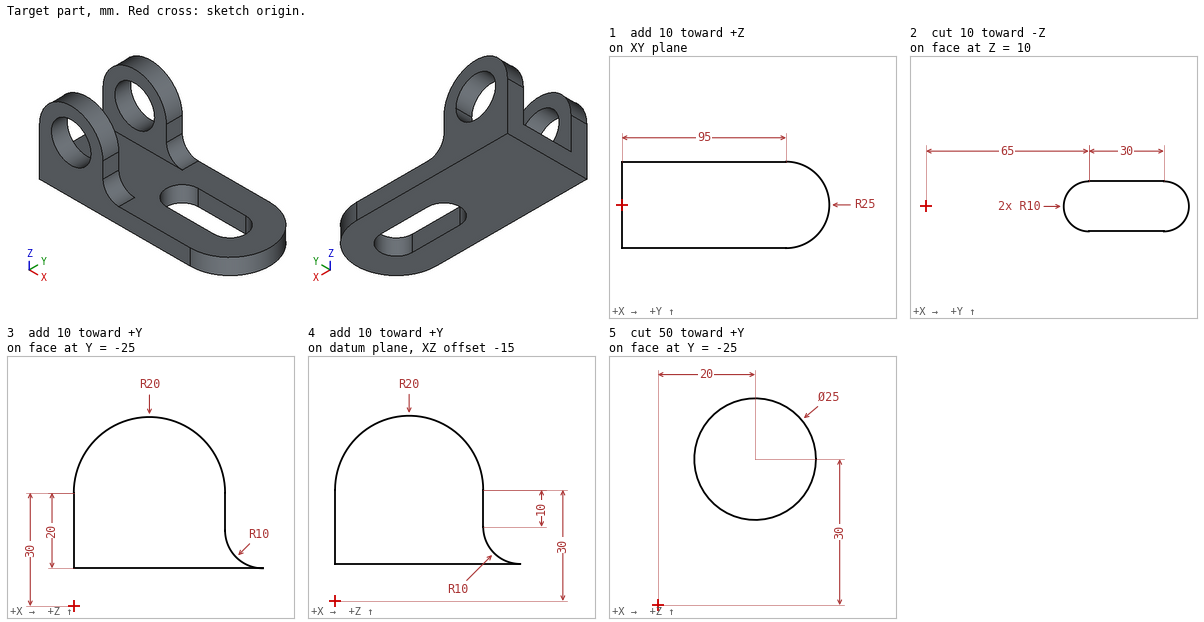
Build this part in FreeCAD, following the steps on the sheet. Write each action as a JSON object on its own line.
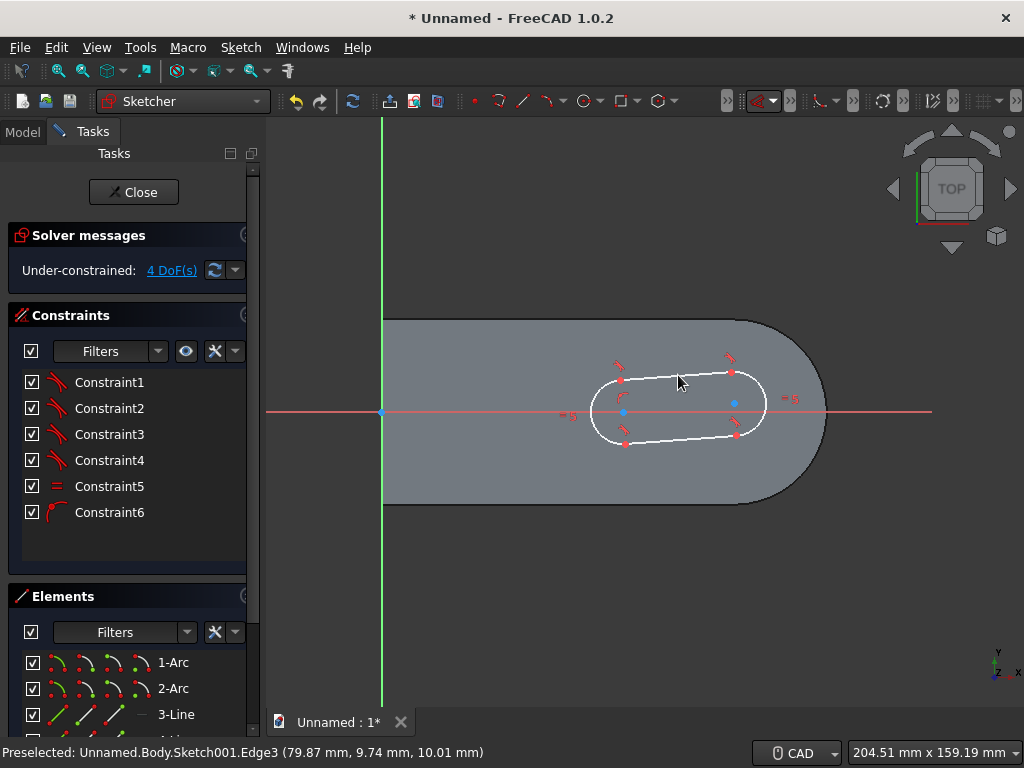
{"action": "left_click", "coordinate": [654, 378]}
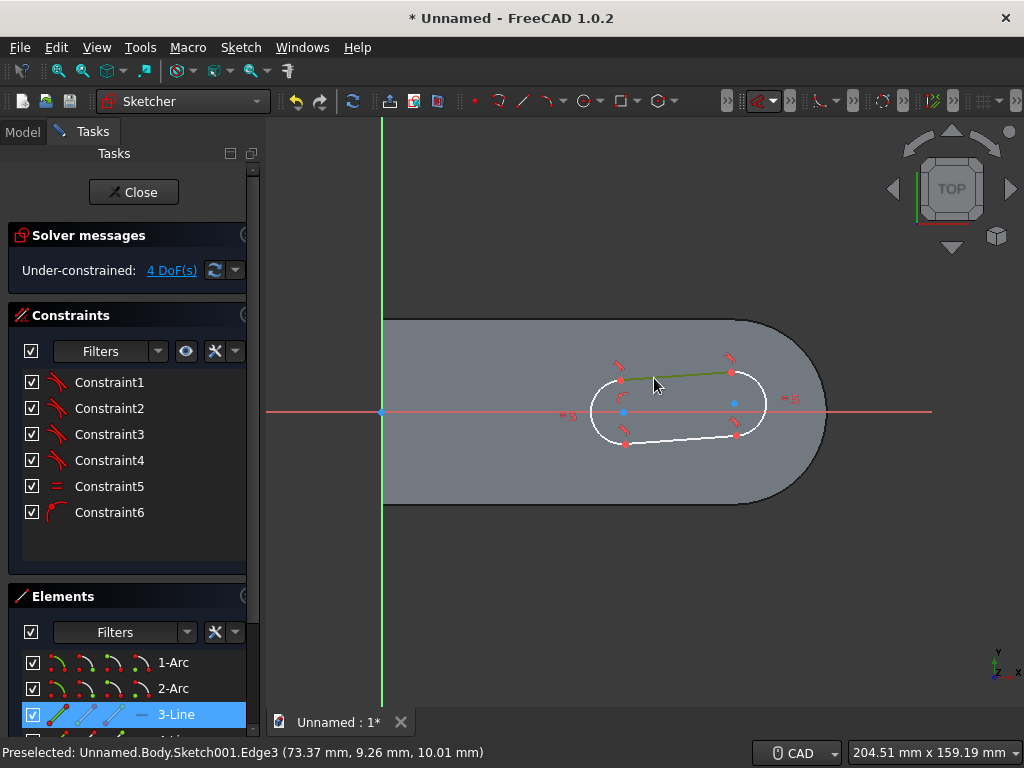
{"action": "key", "text": "h"}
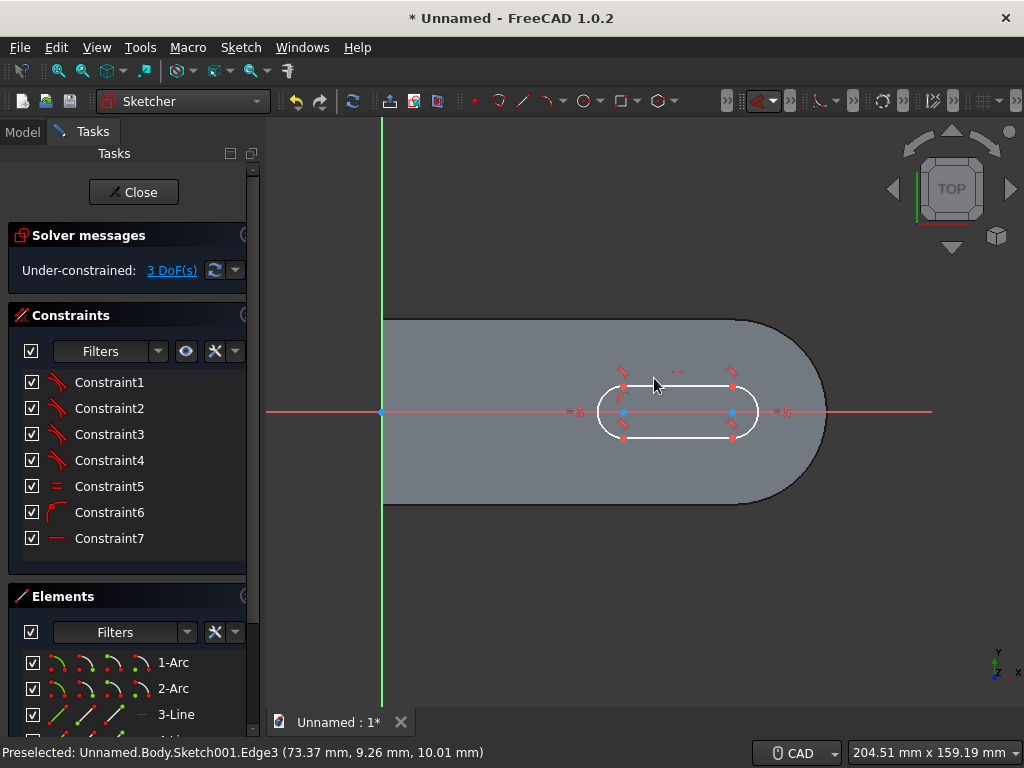
{"action": "left_click", "coordinate": [603, 397]}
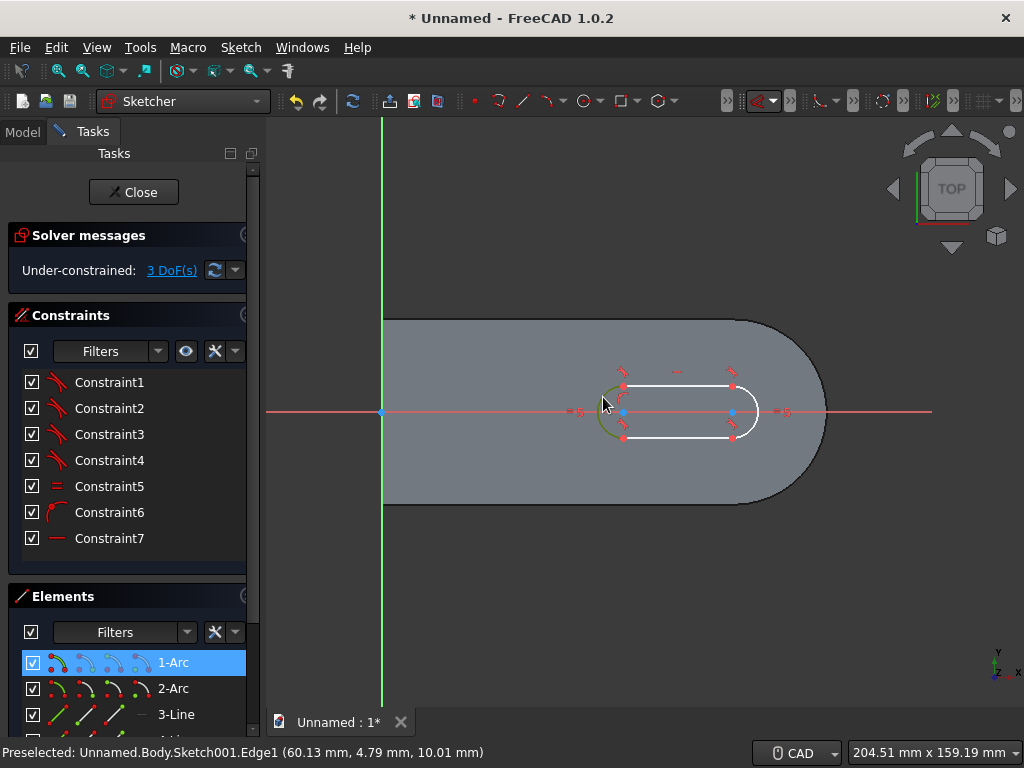
{"action": "left_click", "coordinate": [776, 102]}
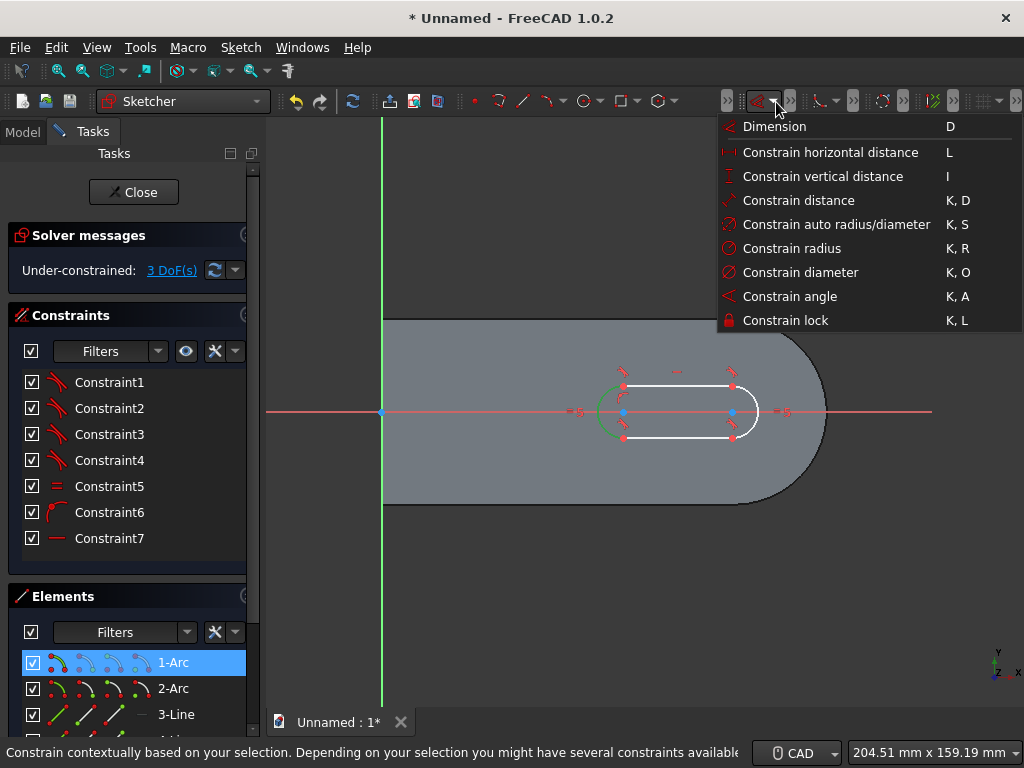
{"action": "left_click", "coordinate": [870, 248]}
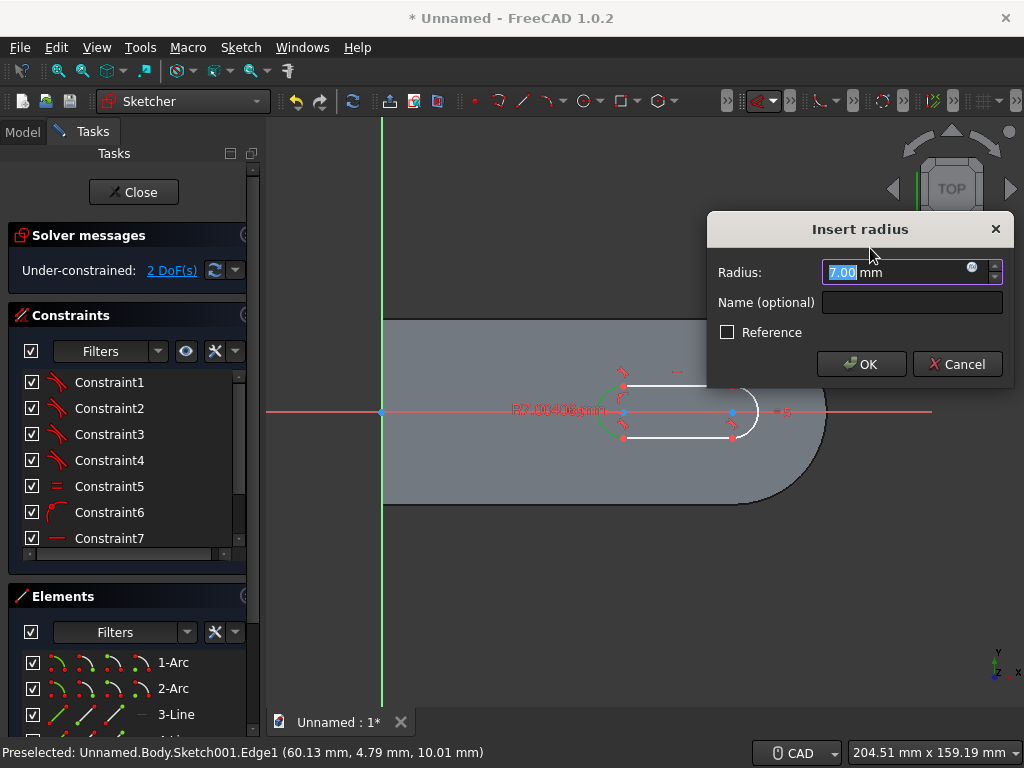
{"action": "type", "text": "10"}
{"action": "key", "text": "Return"}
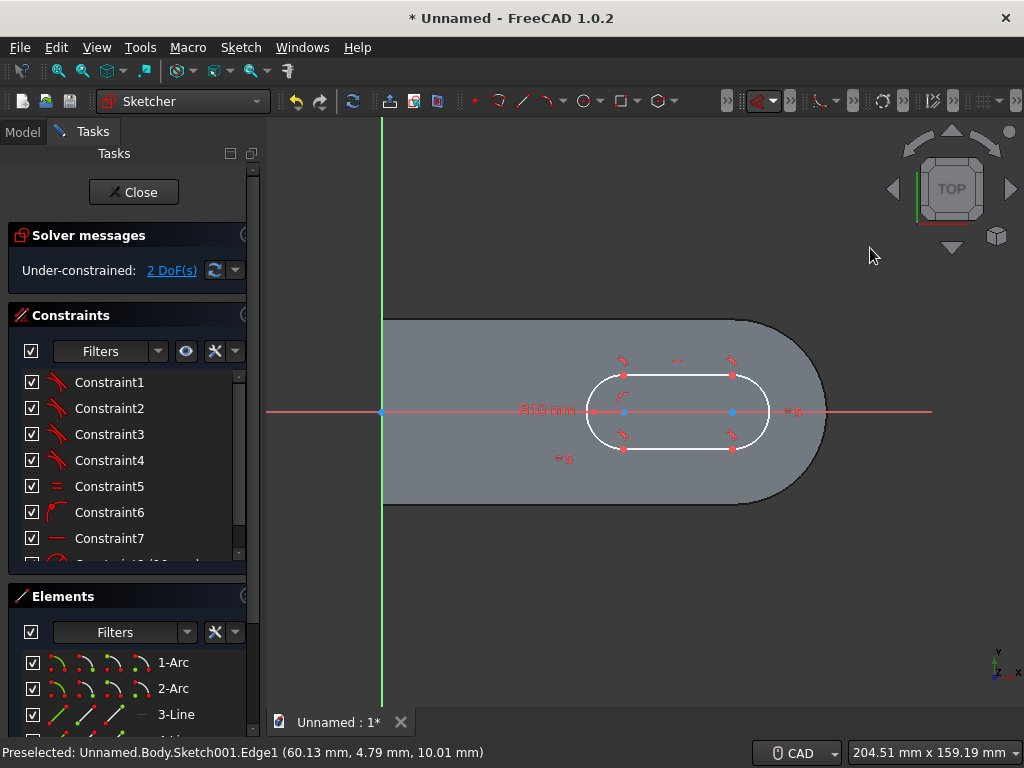
{"action": "left_click", "coordinate": [656, 375]}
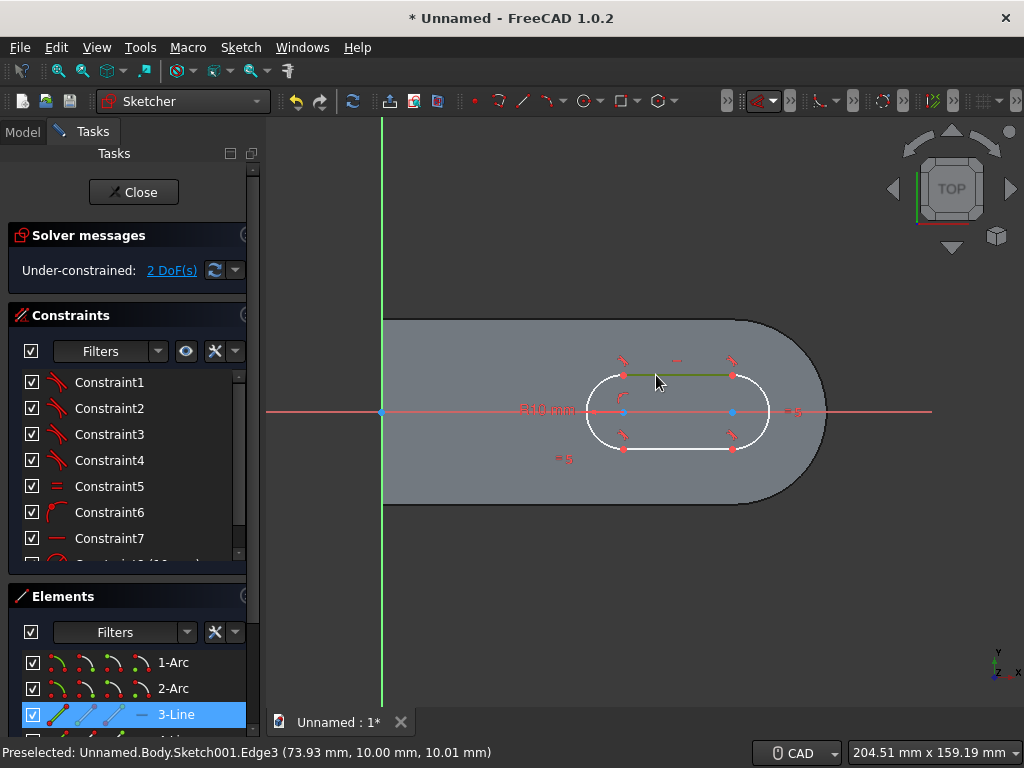
{"action": "left_click", "coordinate": [776, 102]}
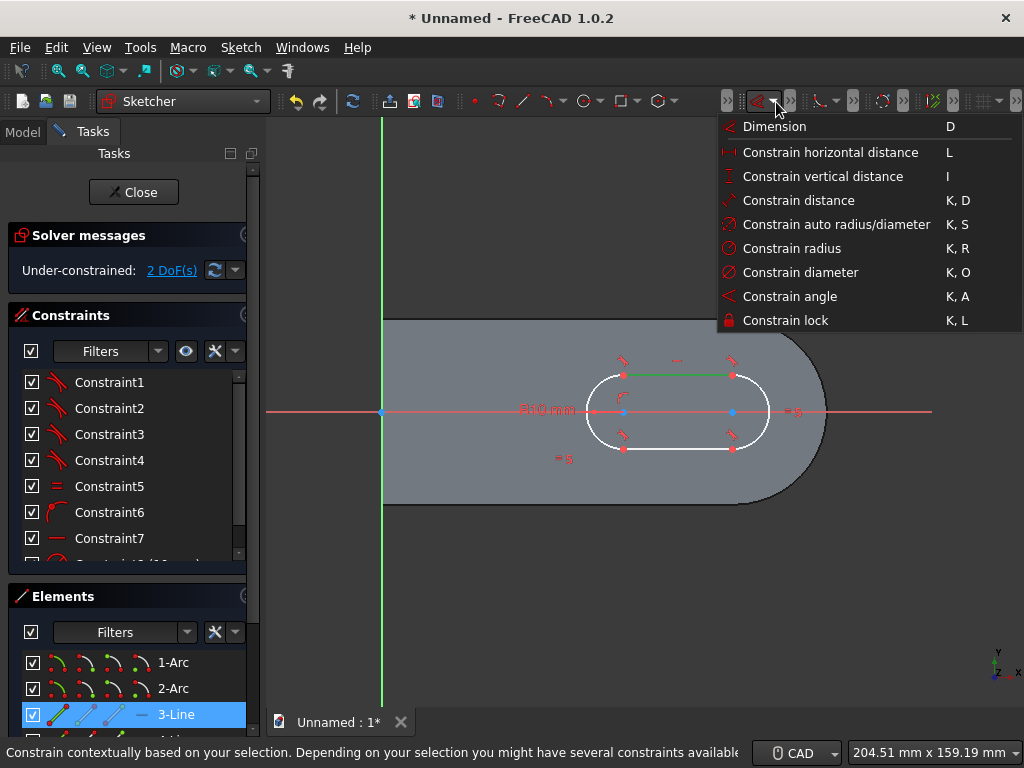
{"action": "left_click", "coordinate": [870, 152]}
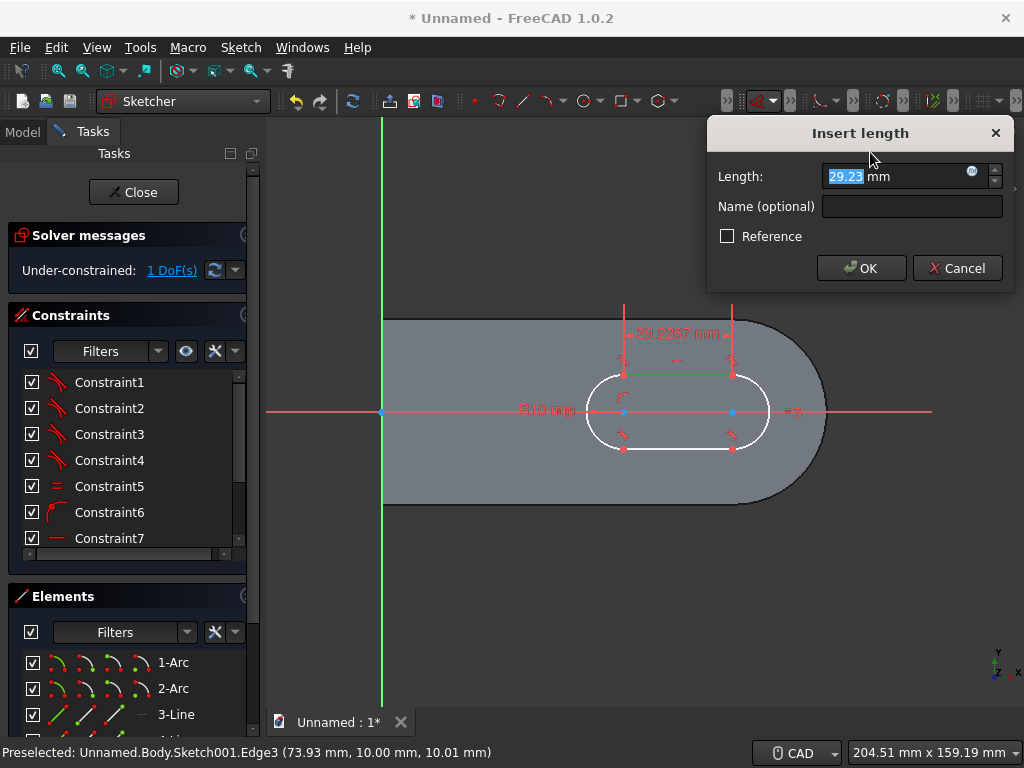
{"action": "type", "text": "30"}
{"action": "key", "text": "Return"}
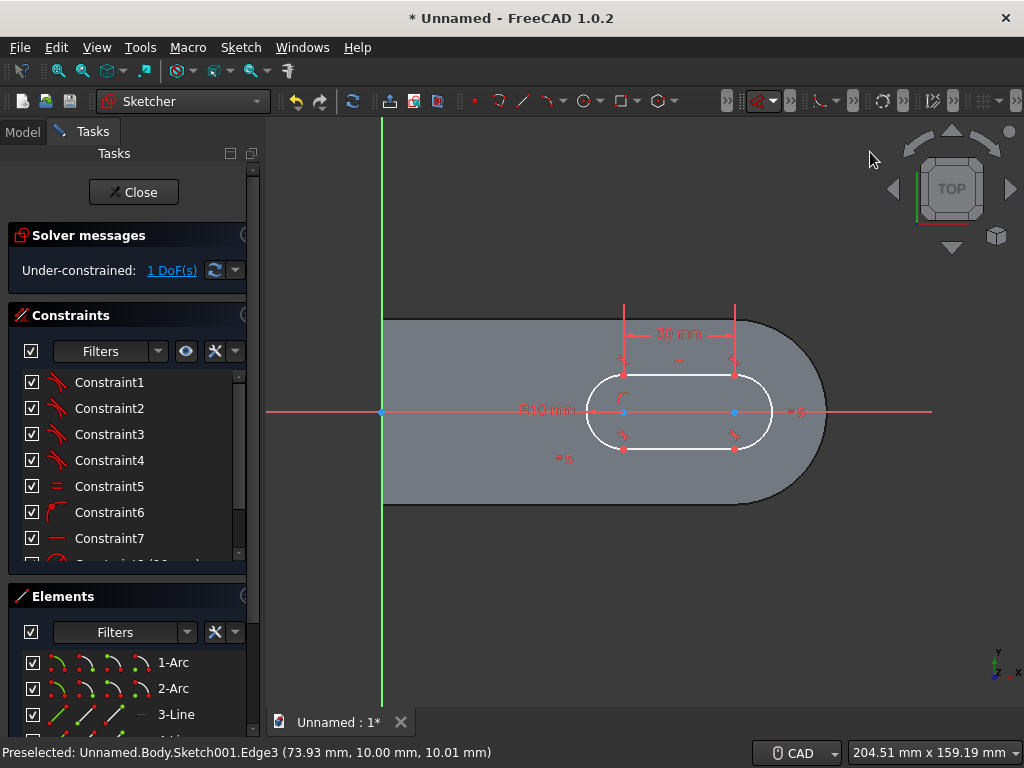
{"action": "left_click", "coordinate": [624, 375]}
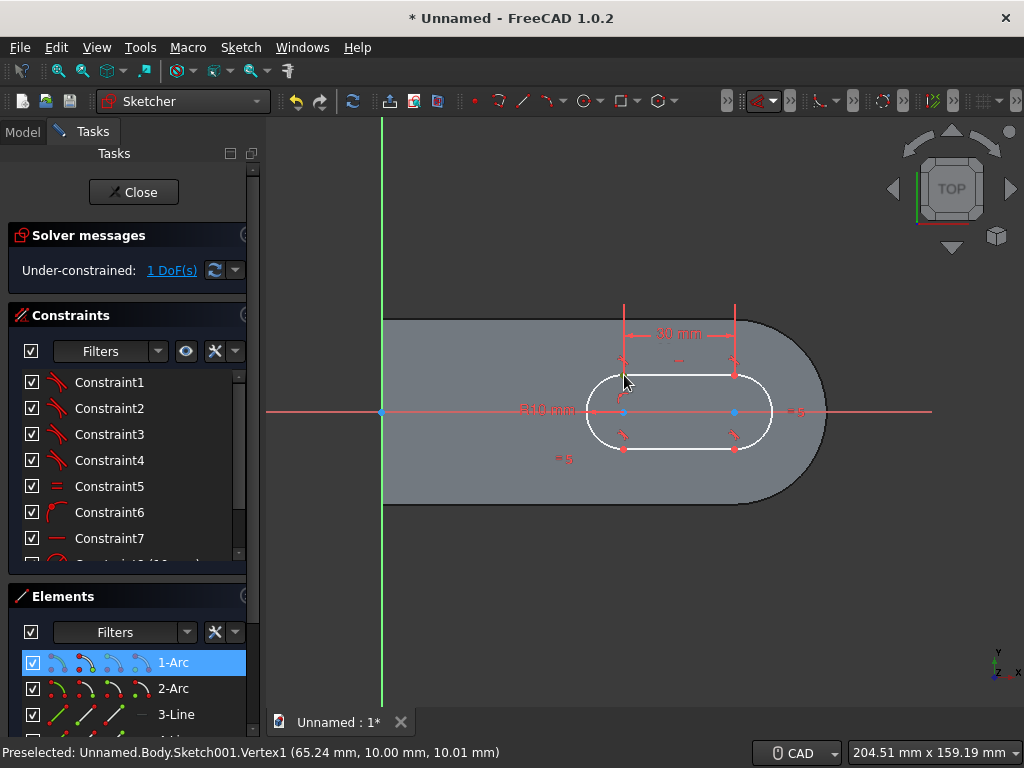
{"action": "left_click", "coordinate": [776, 102]}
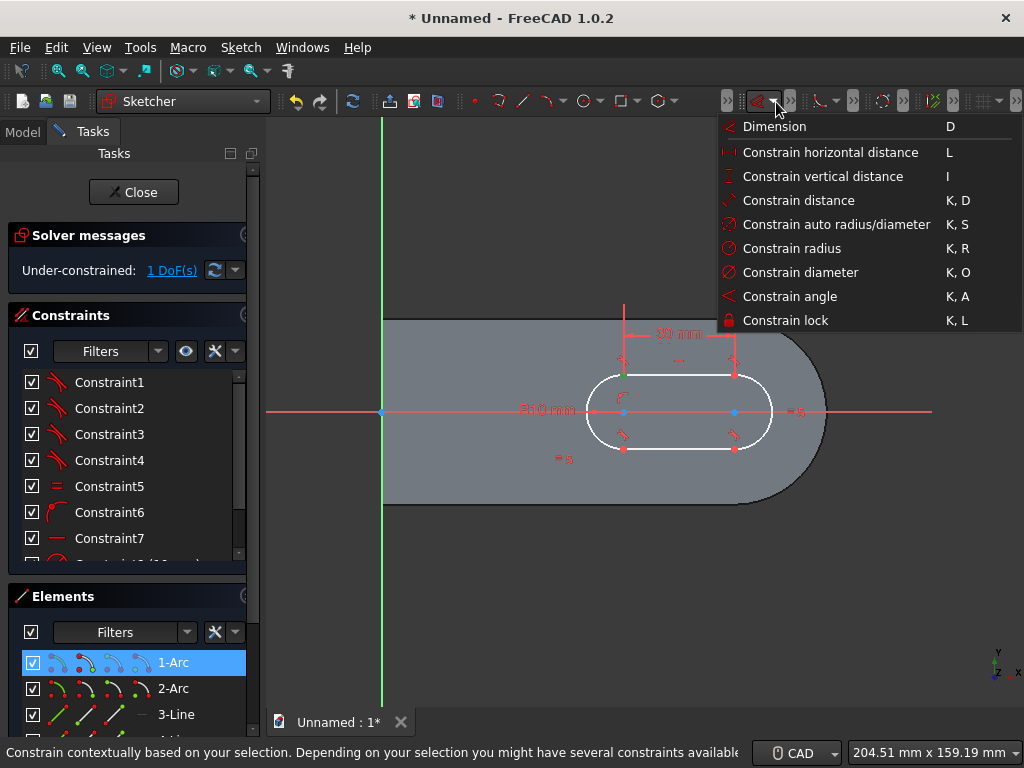
{"action": "left_click", "coordinate": [870, 152]}